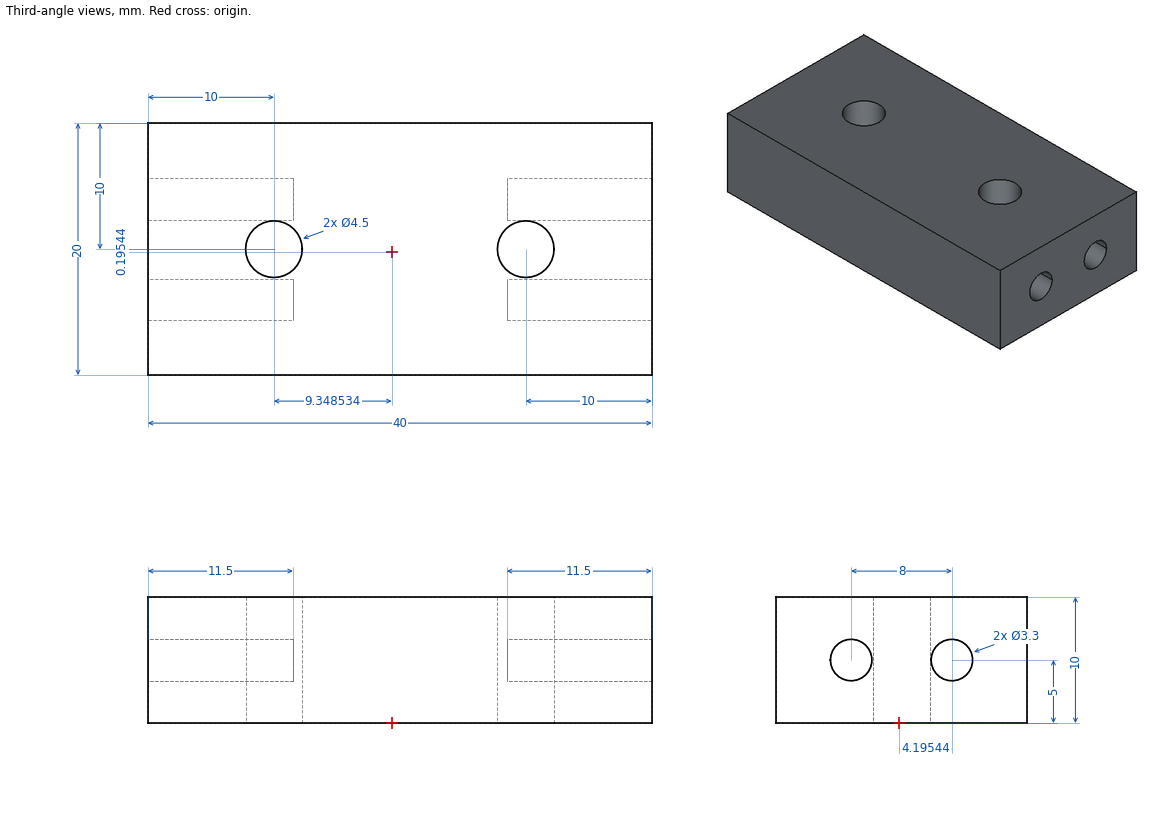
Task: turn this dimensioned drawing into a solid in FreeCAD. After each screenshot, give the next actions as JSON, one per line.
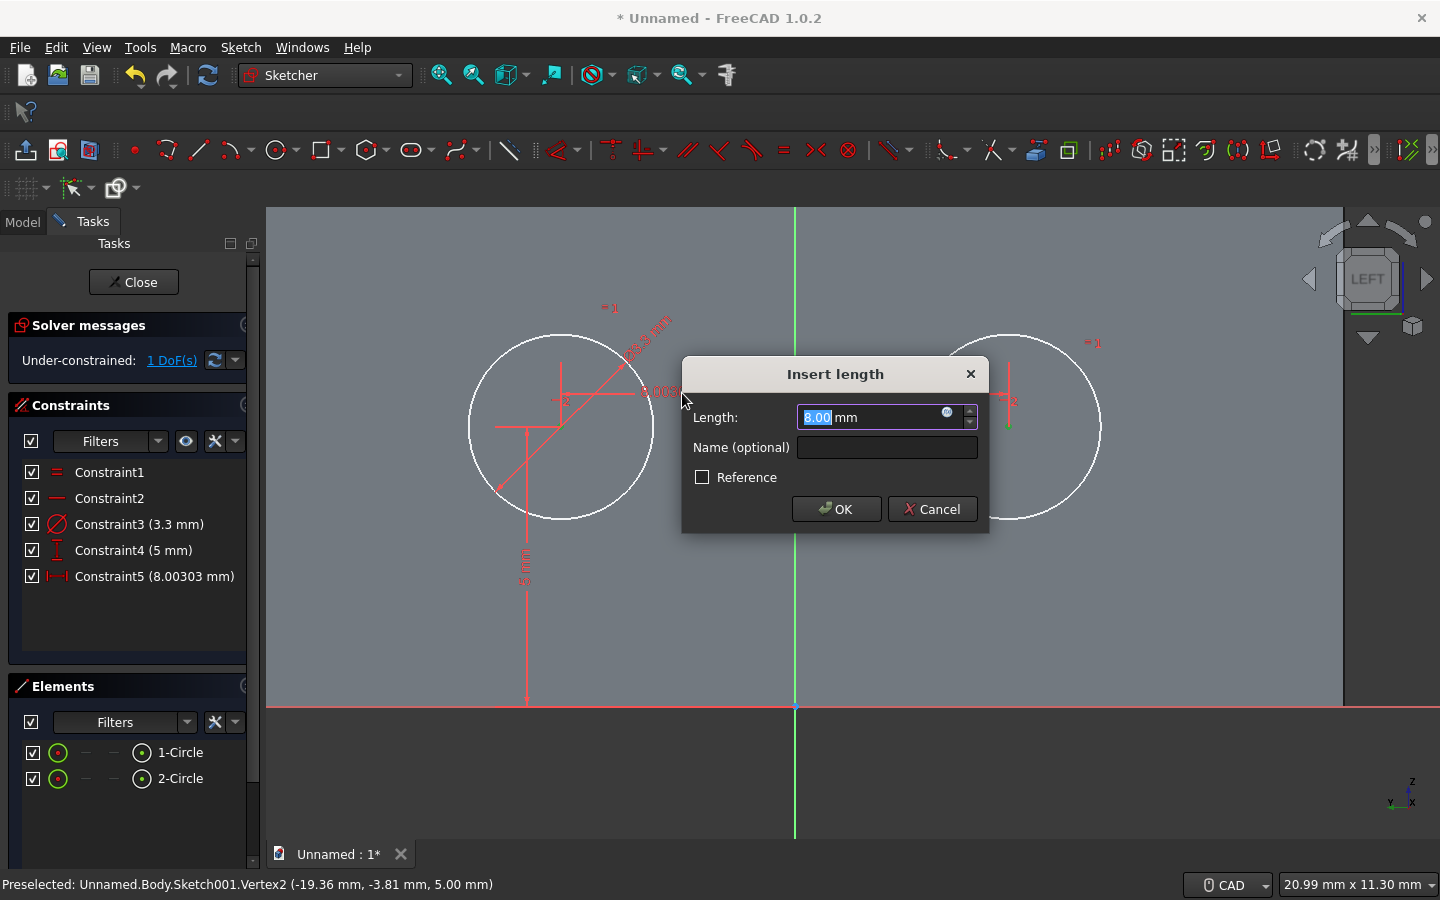
{"action": "type", "text": "8"}
{"action": "key", "text": "Return"}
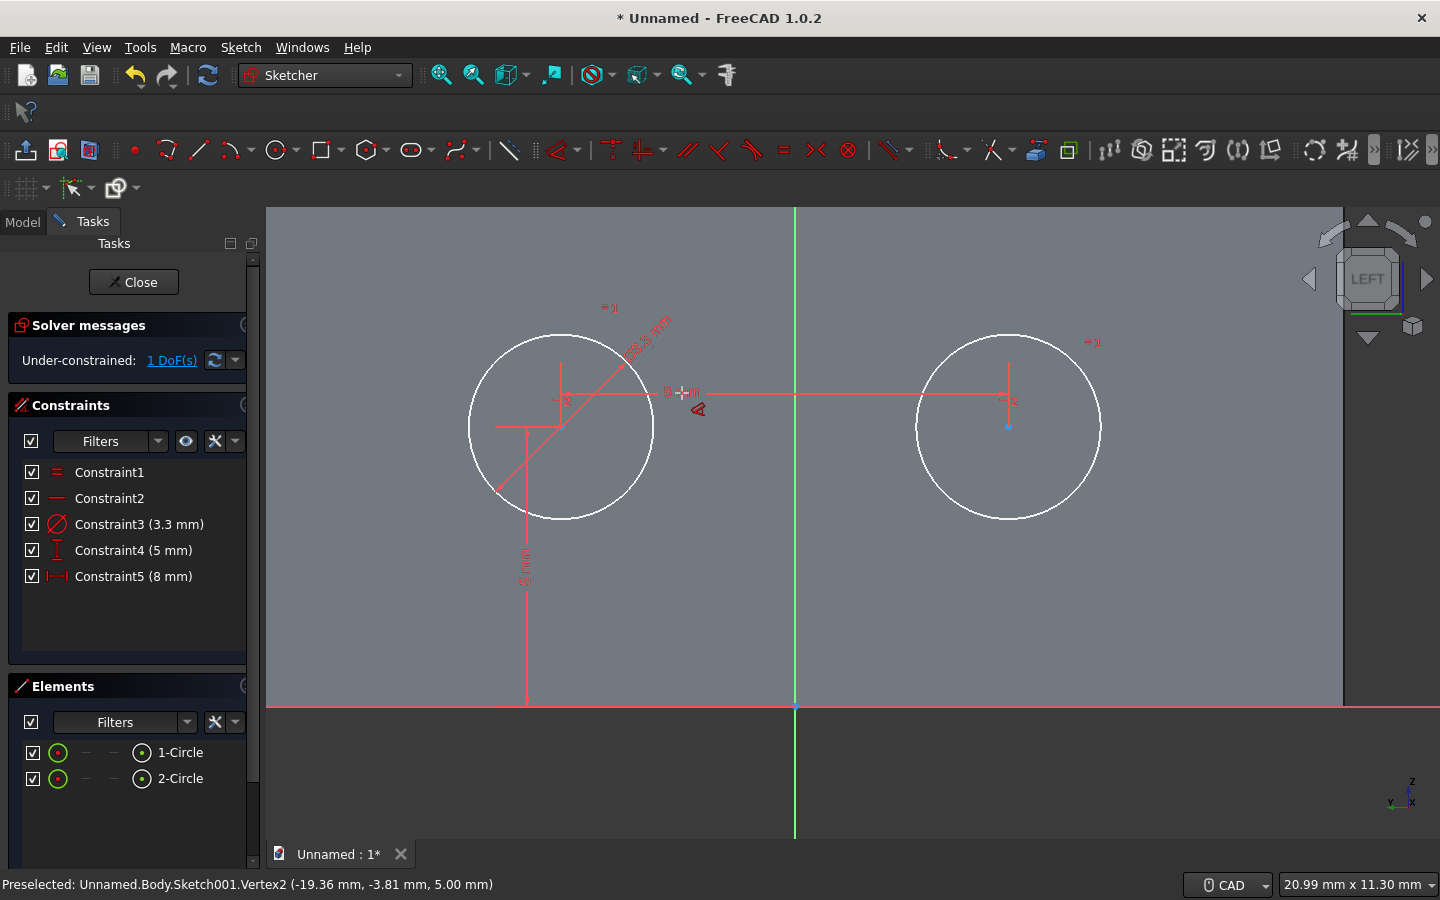
{"action": "left_click", "coordinate": [561, 427]}
{"action": "left_click", "coordinate": [678, 741]}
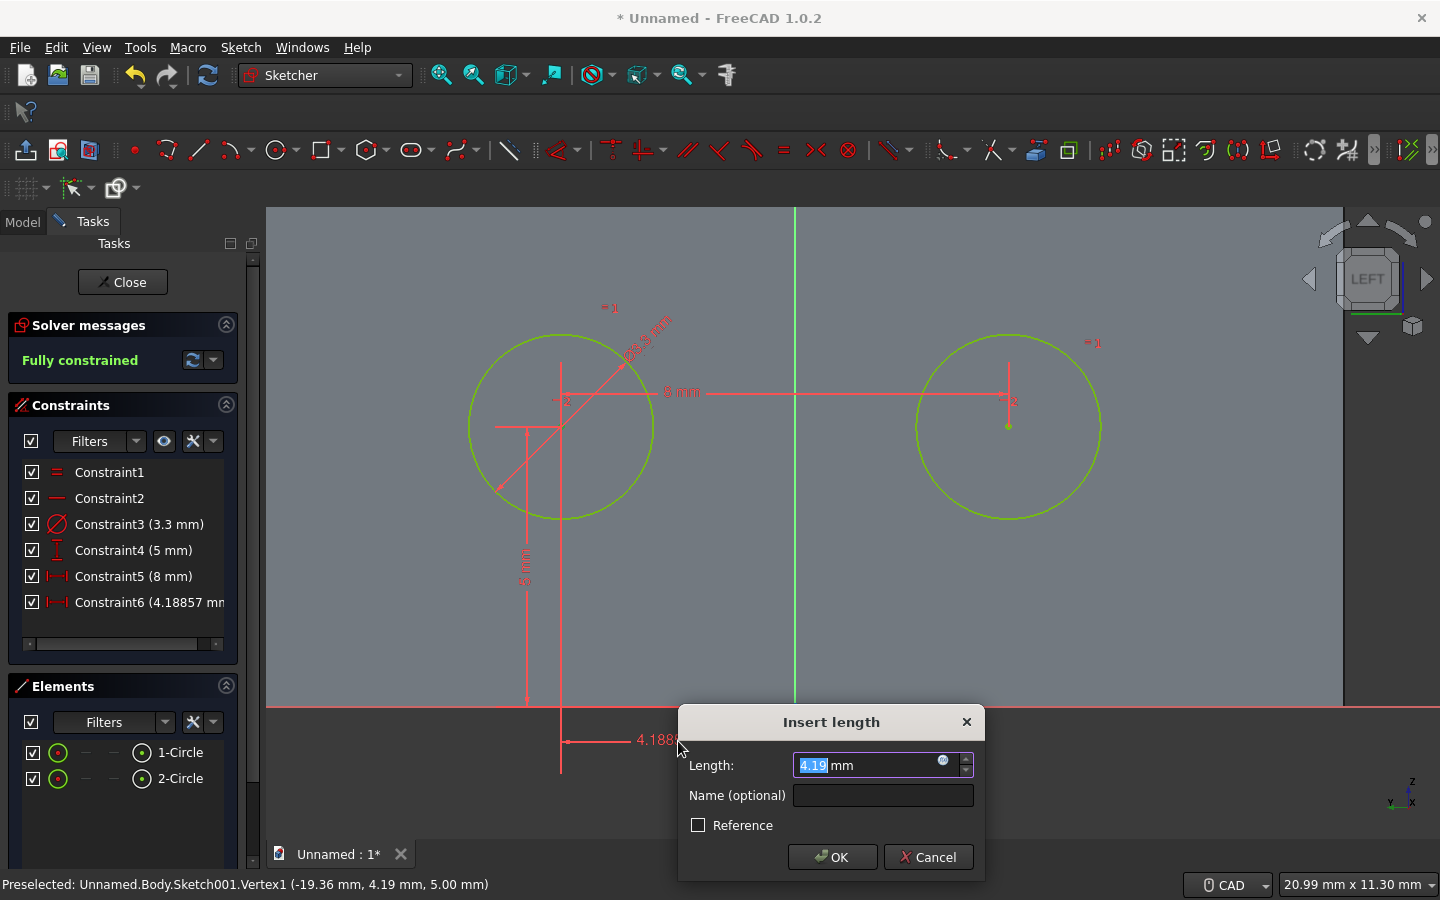
{"action": "type", "text": "4.19544"}
{"action": "key", "text": "Return"}
{"action": "key", "text": "Escape"}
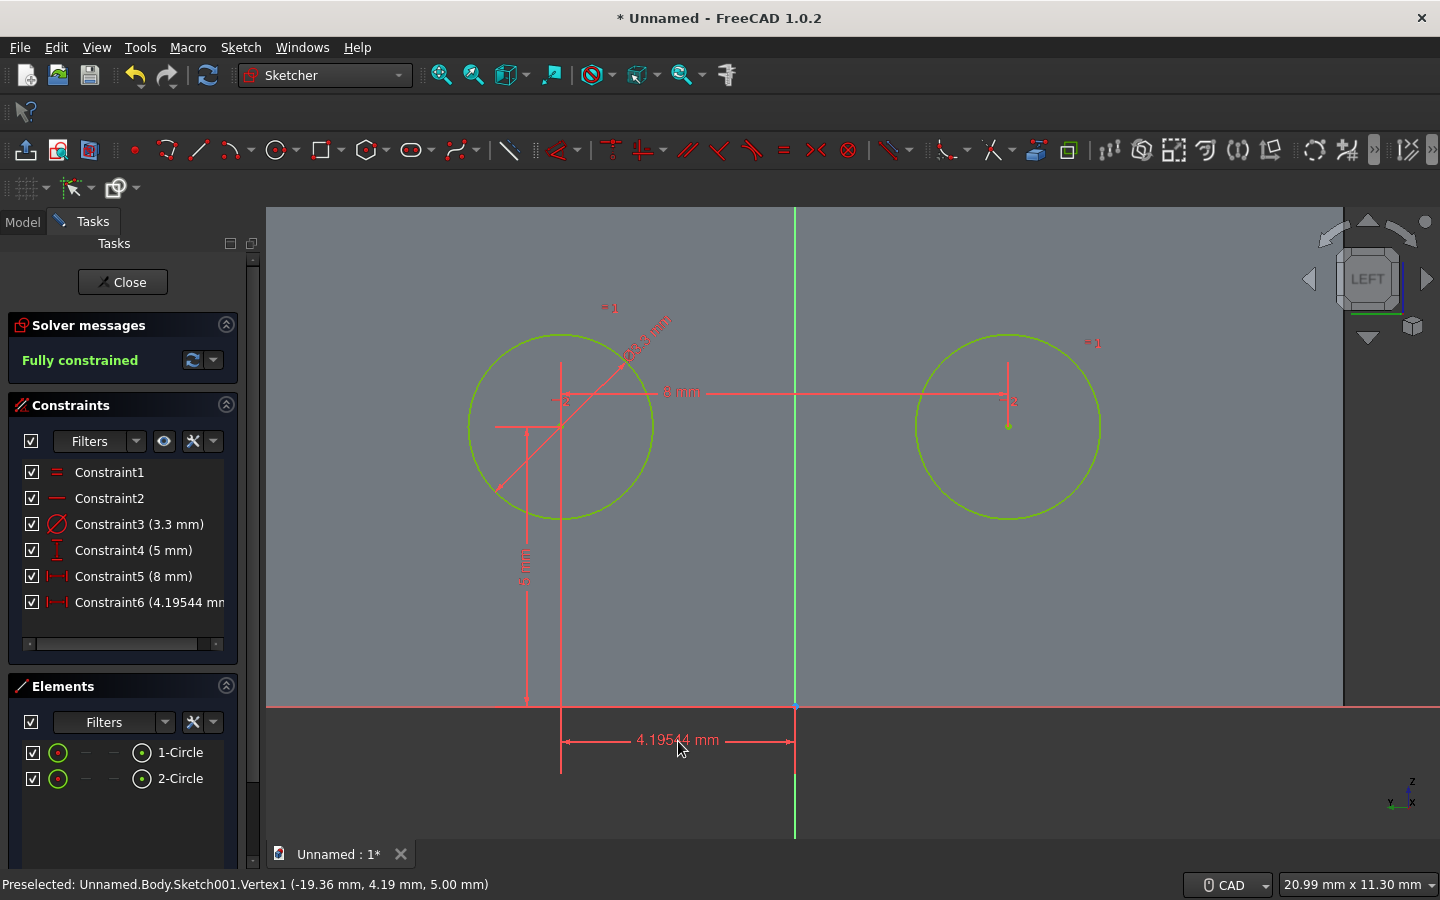
{"action": "left_click", "coordinate": [123, 282]}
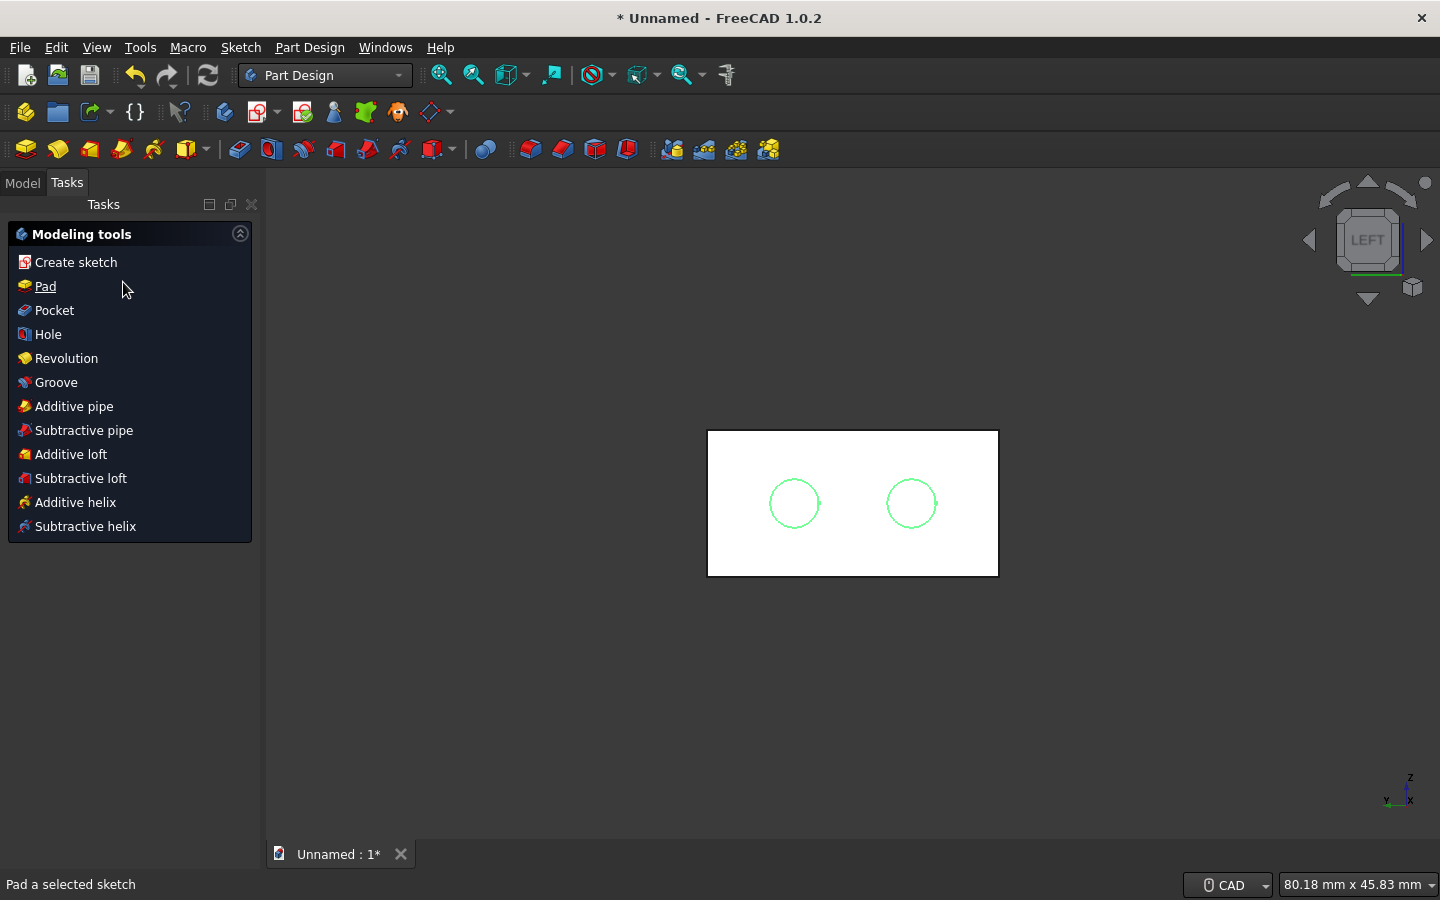
{"action": "left_click", "coordinate": [240, 150]}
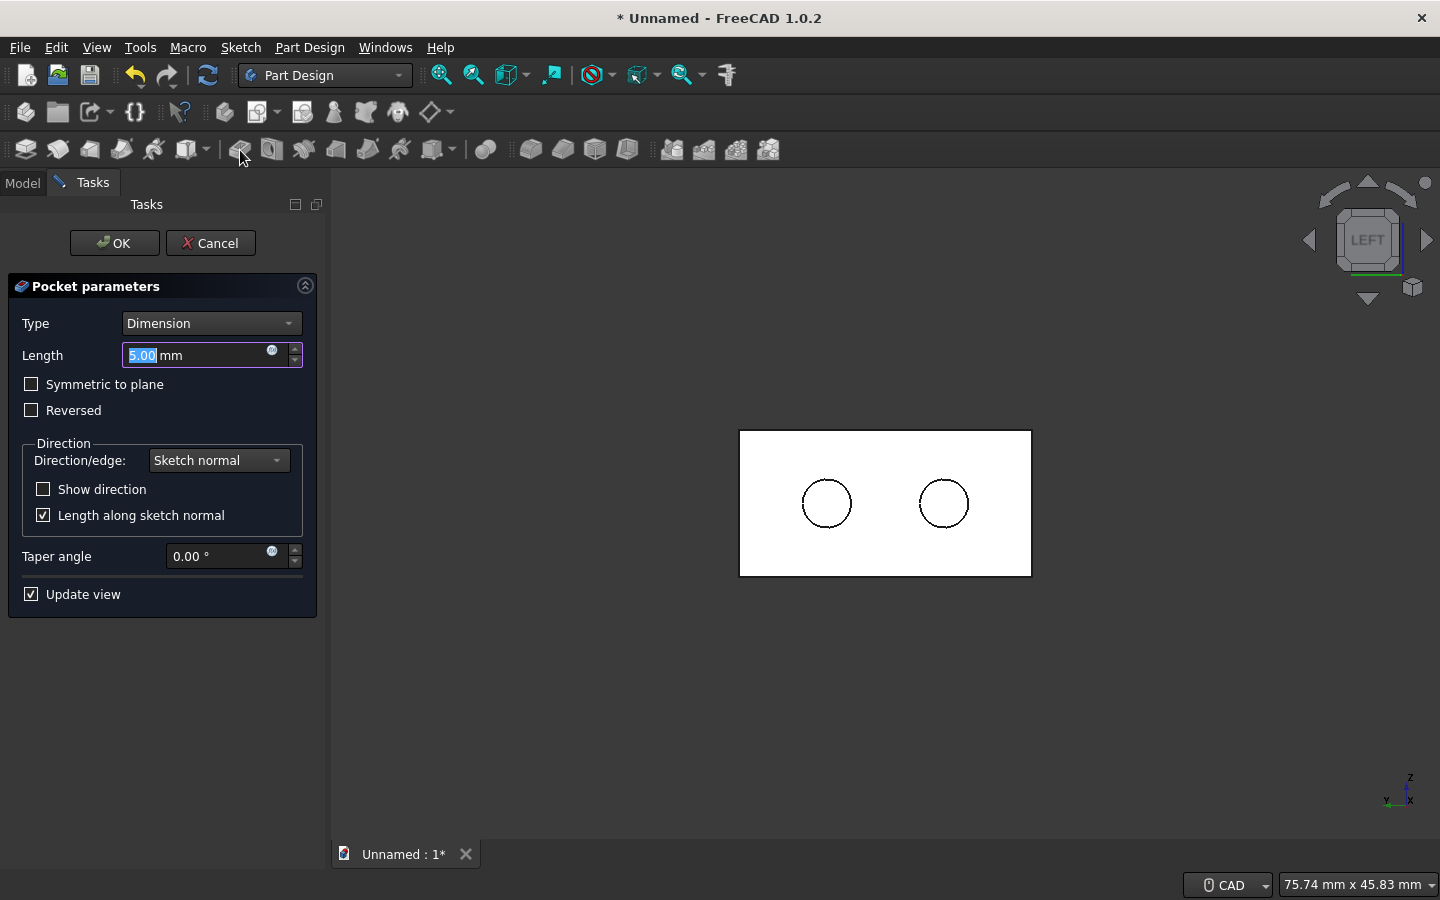
{"action": "type", "text": "11.5"}
{"action": "key", "text": "Tab"}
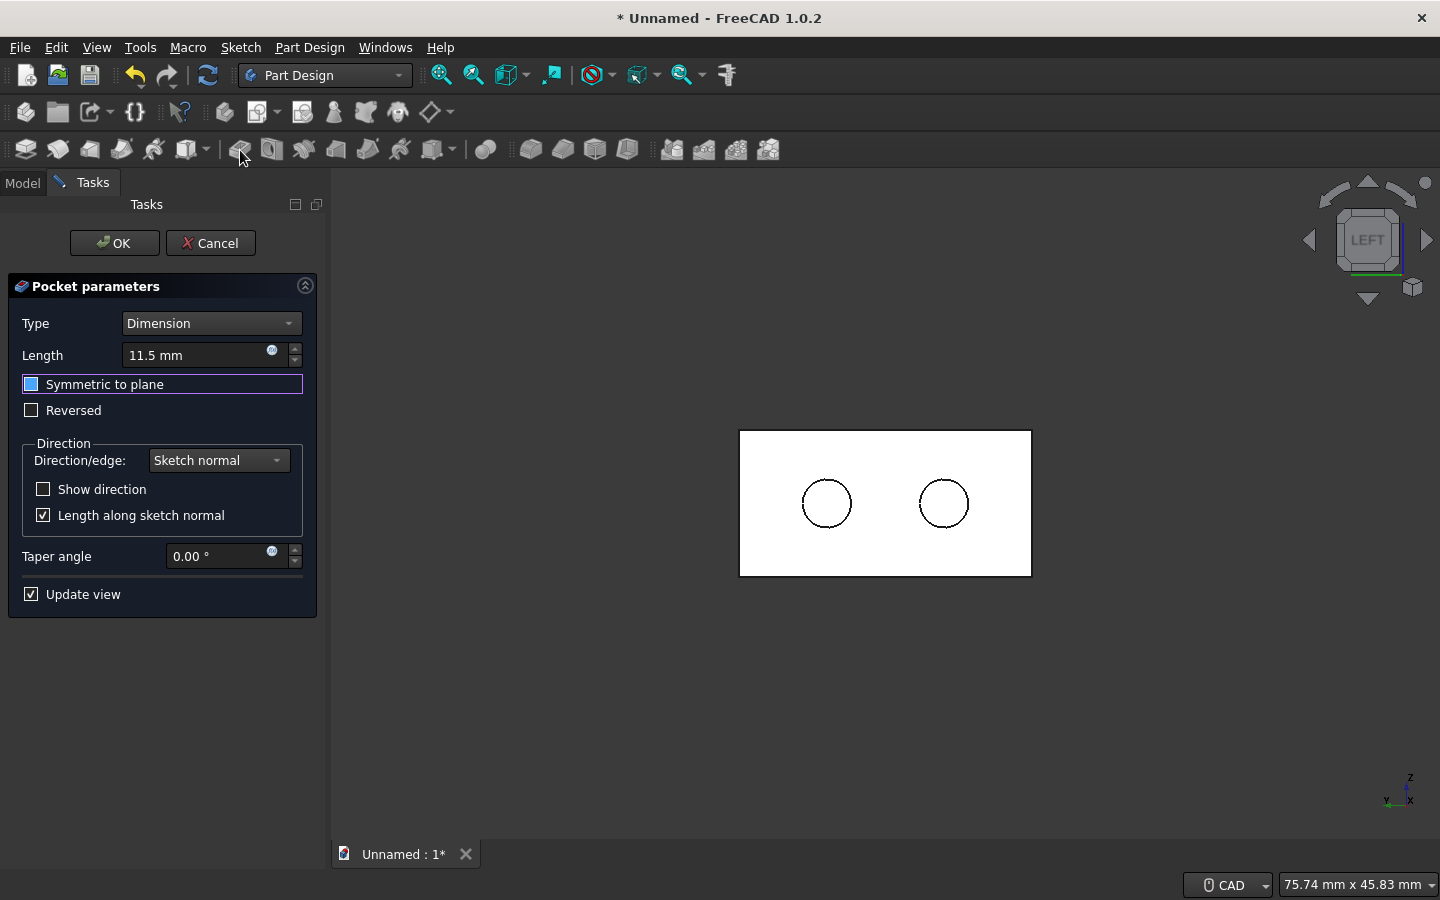
{"action": "left_click", "coordinate": [115, 243]}